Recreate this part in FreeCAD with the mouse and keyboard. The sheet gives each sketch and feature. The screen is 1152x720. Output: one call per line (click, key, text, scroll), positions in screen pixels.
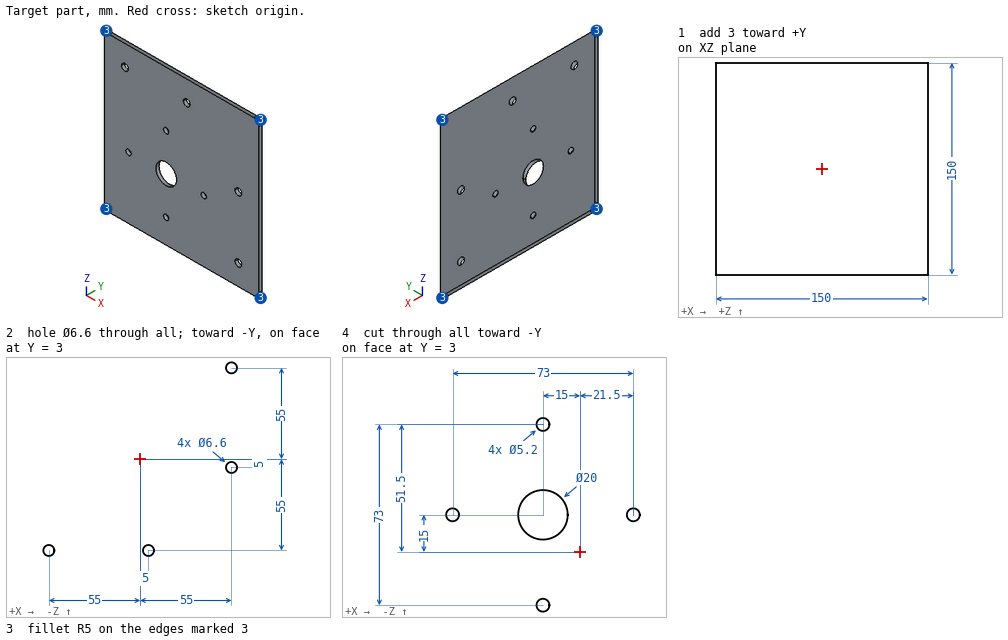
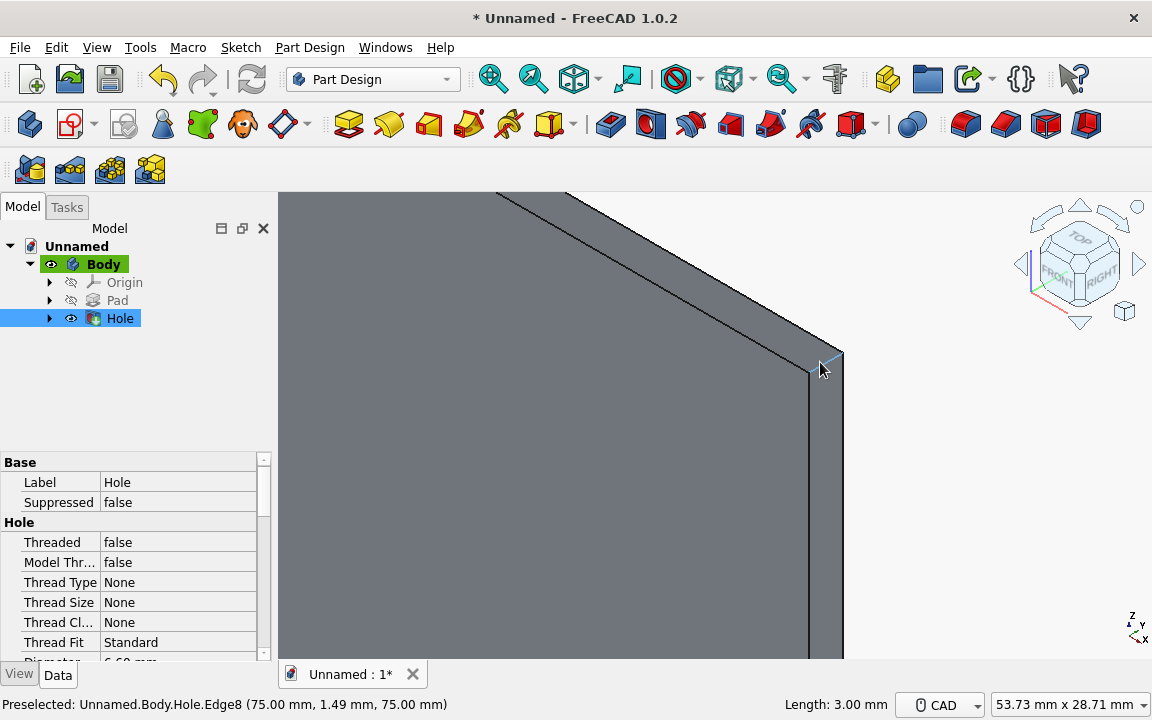
click(494, 80)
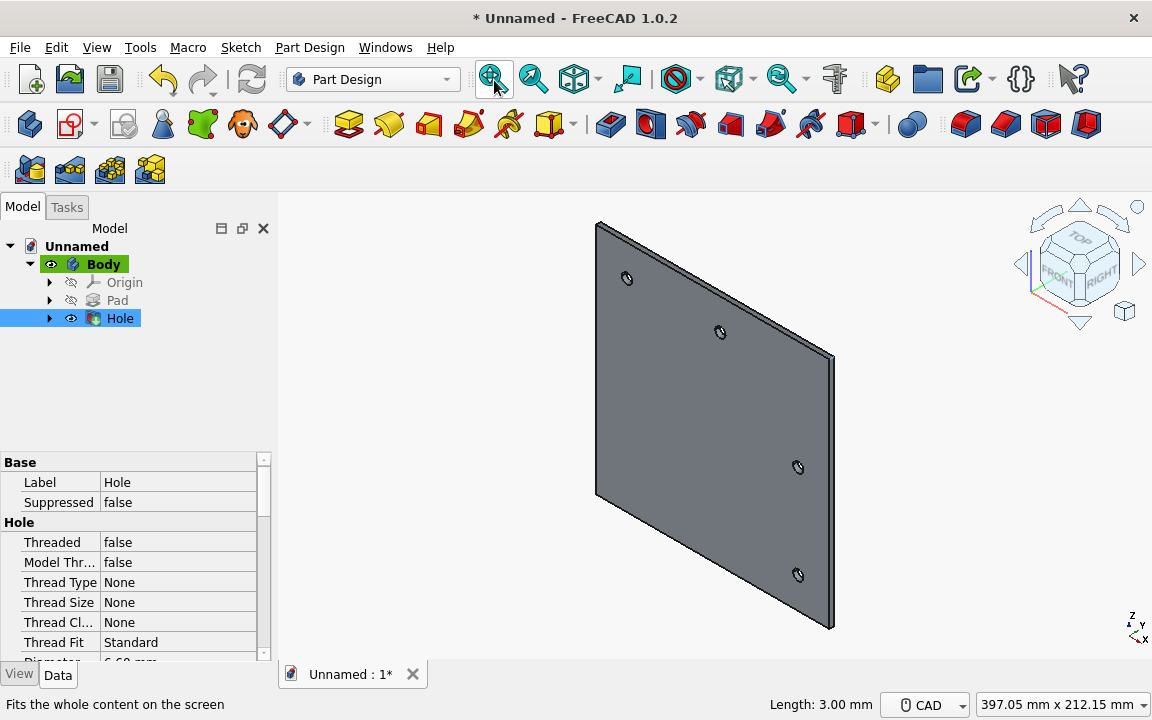
key(2)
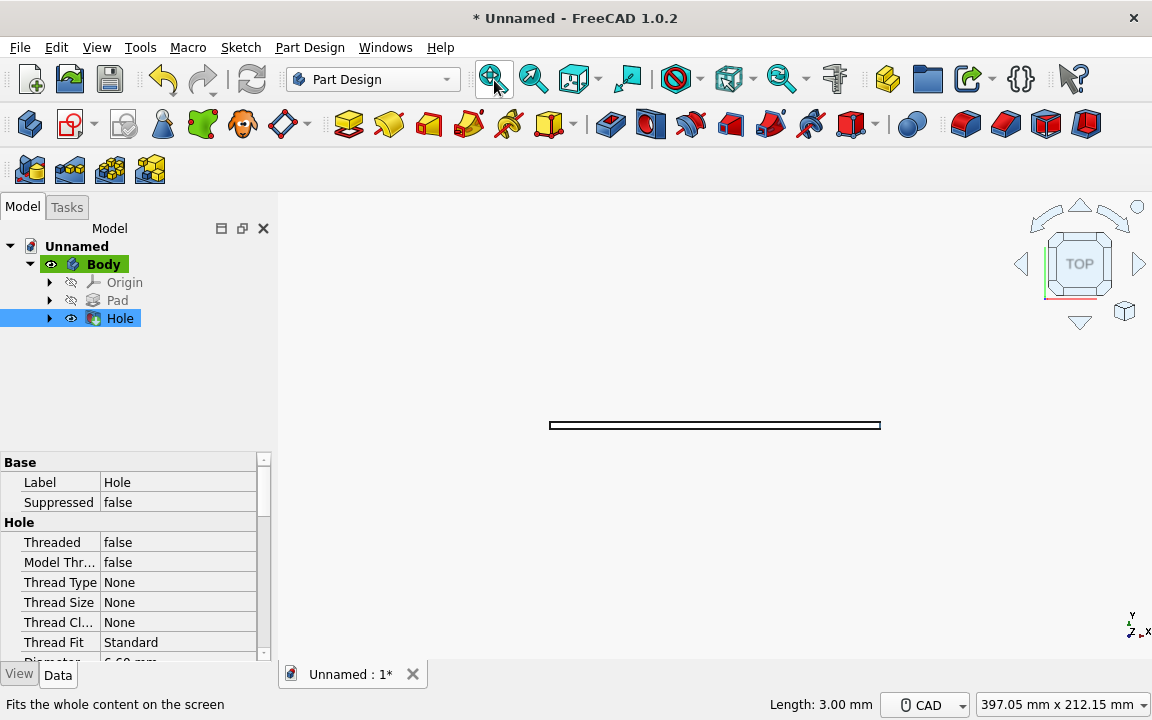
click(494, 80)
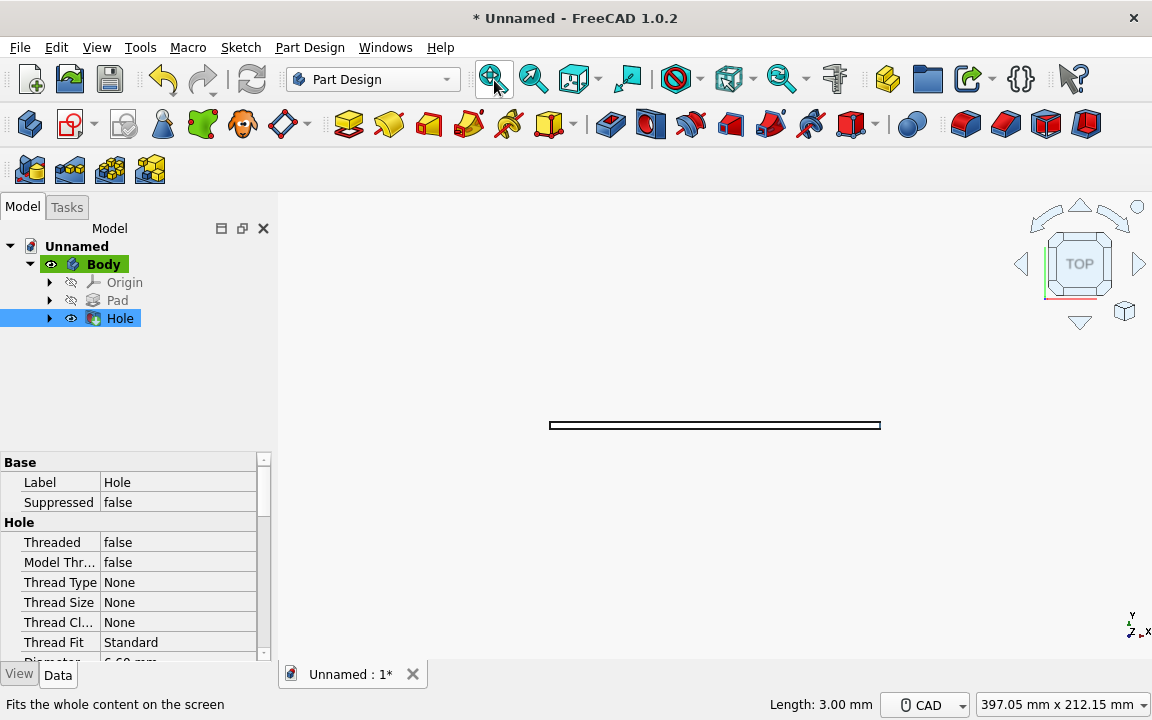
scroll(550, 424, up, 10)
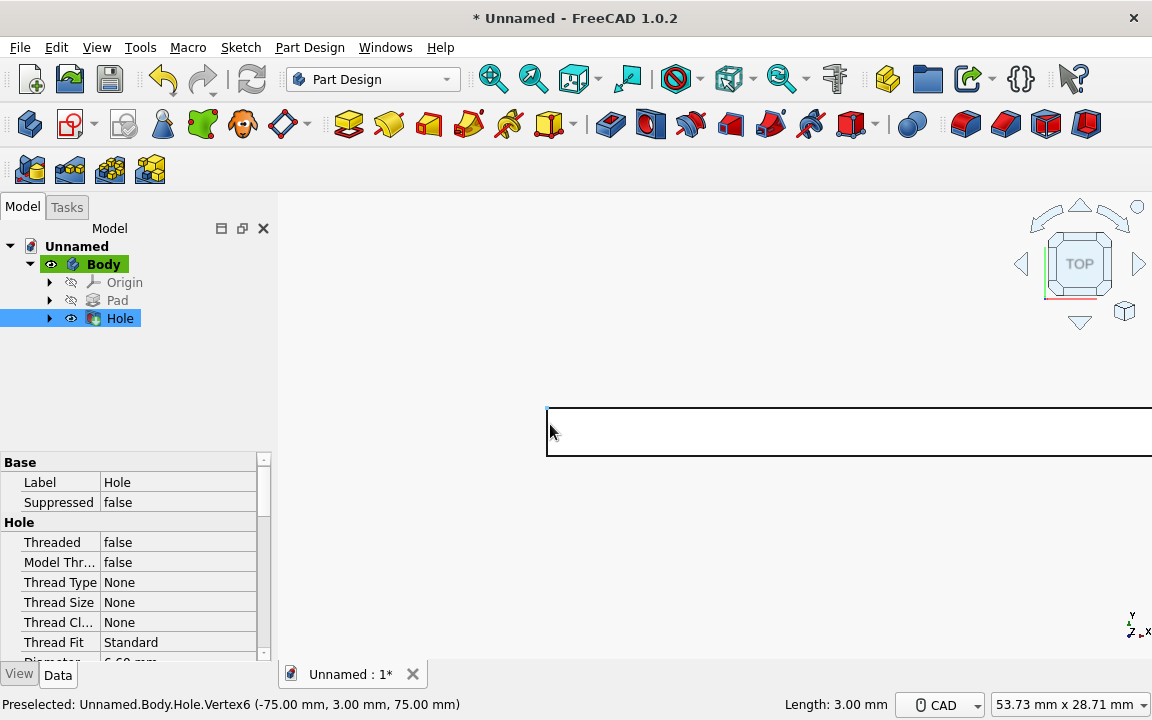
click(547, 431, ctrl)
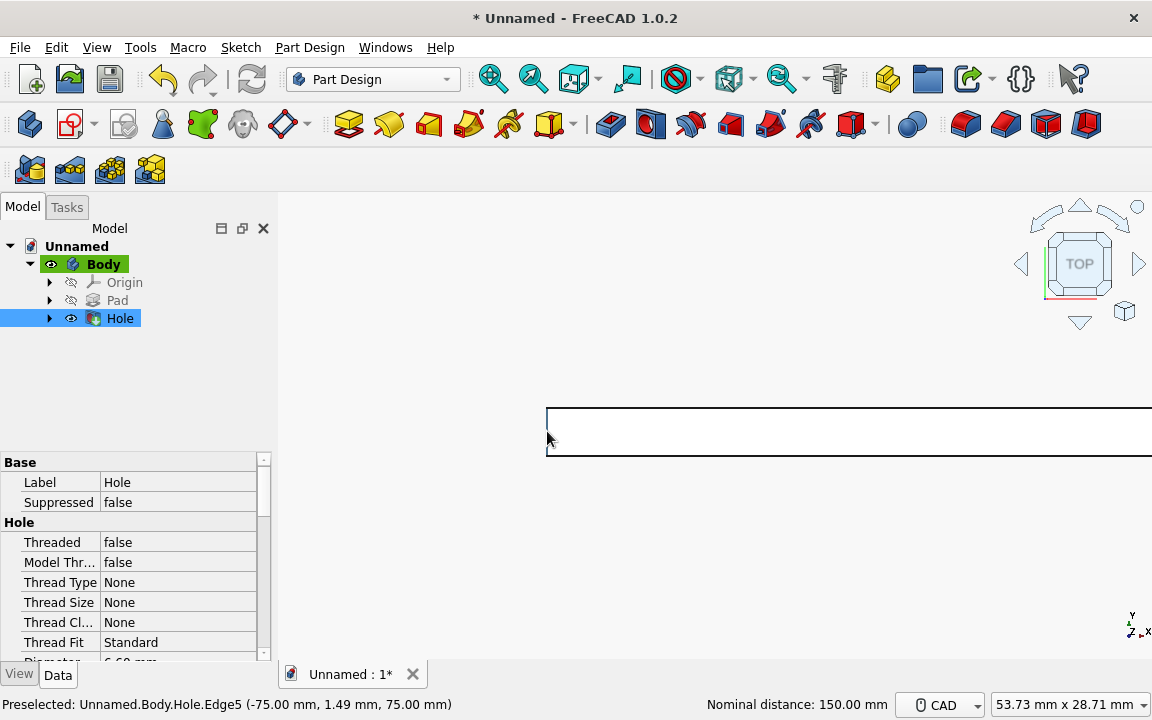
click(494, 80)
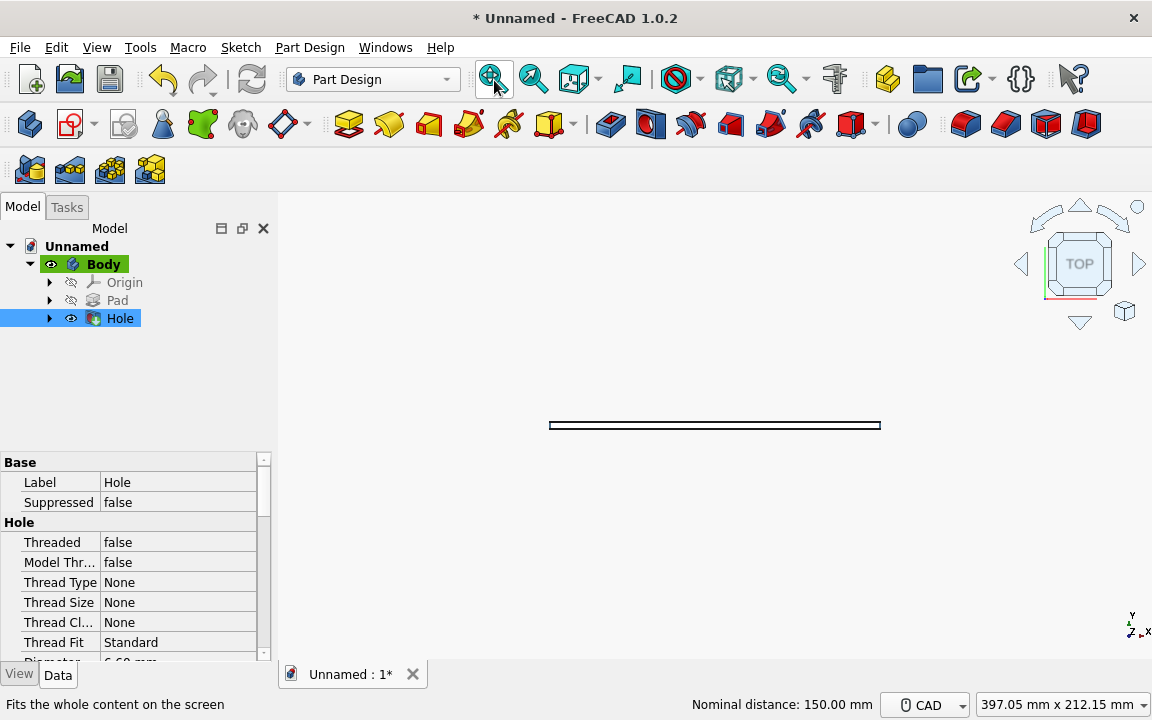
key(1)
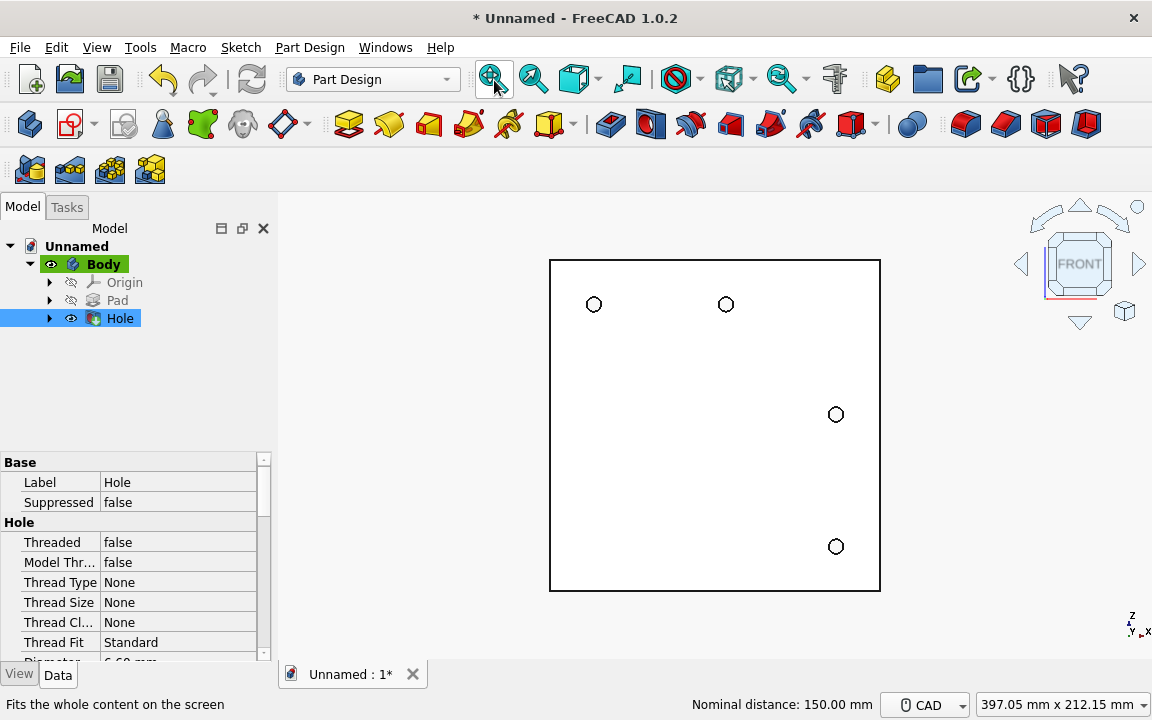
scroll(550, 590, up, 10)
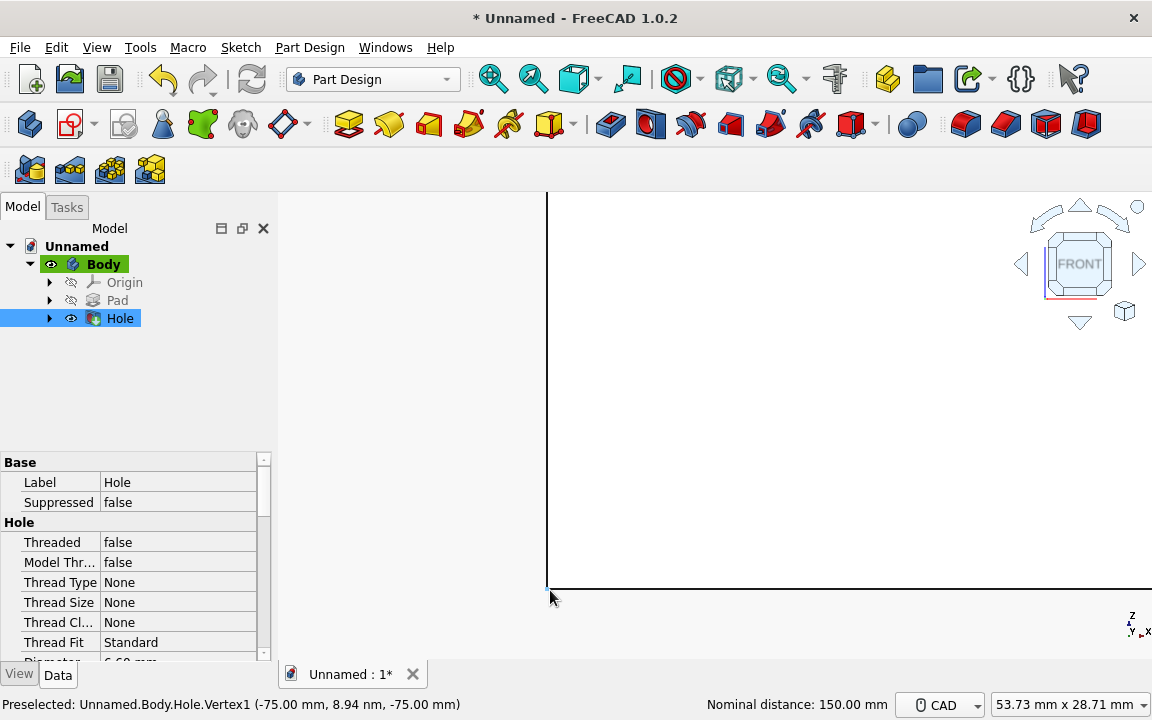
click(494, 80)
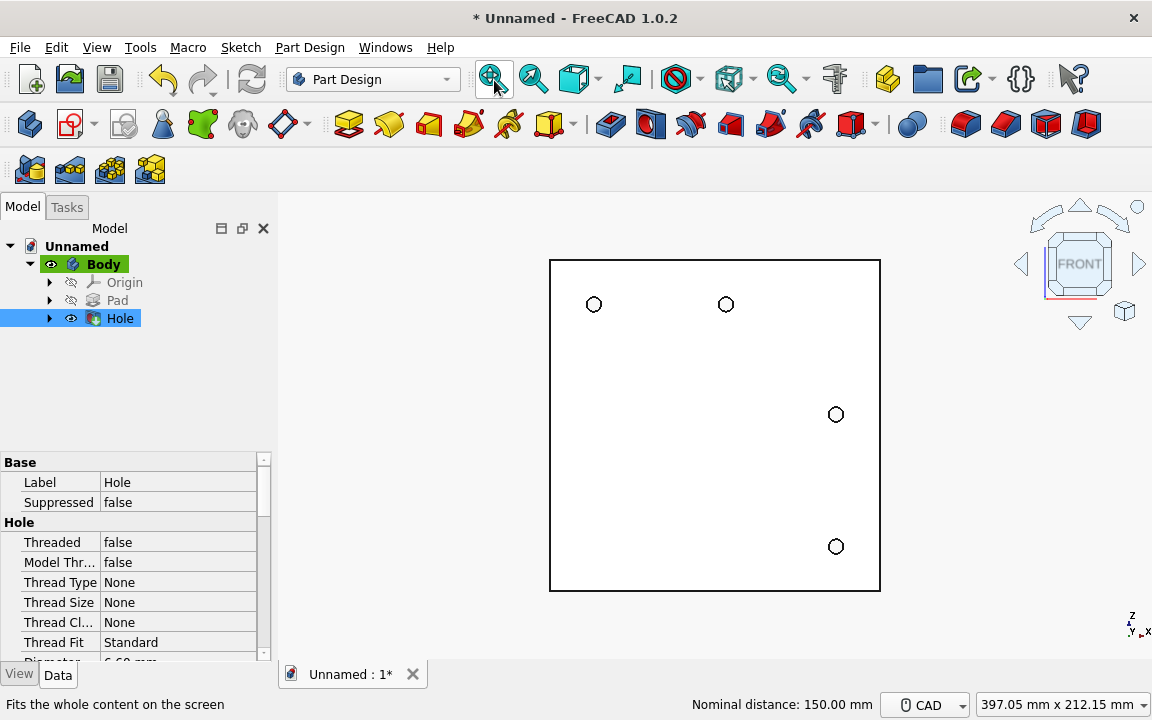
key(3)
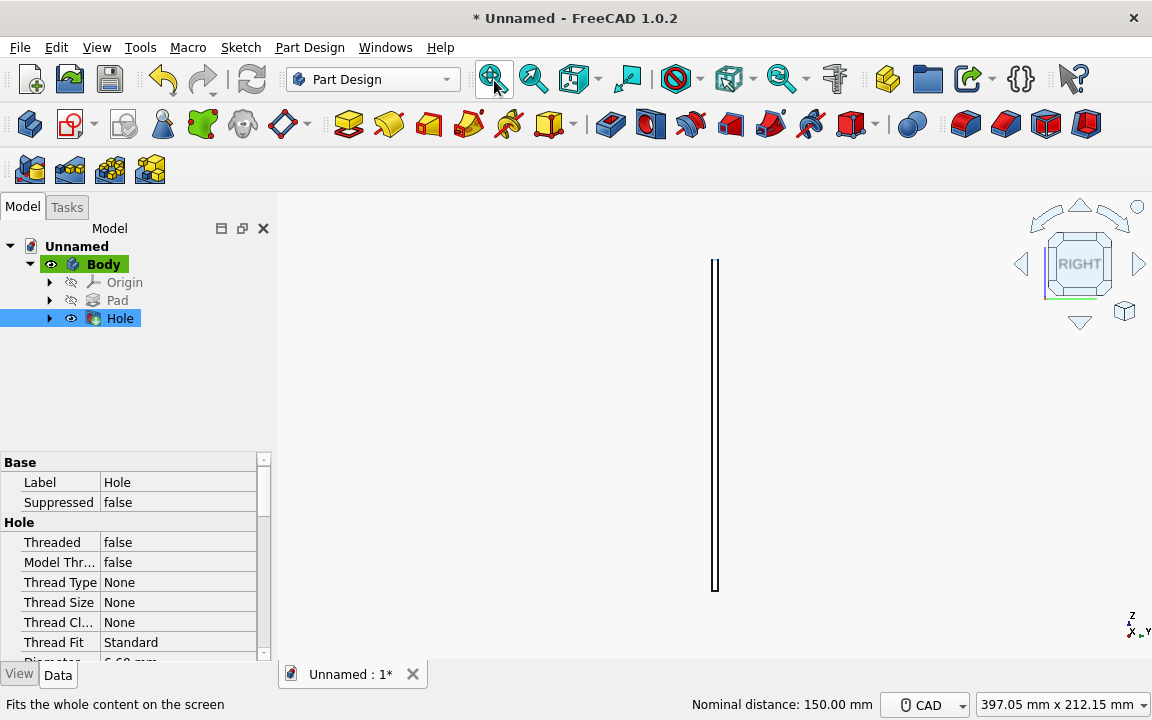
scroll(715, 590, up, 10)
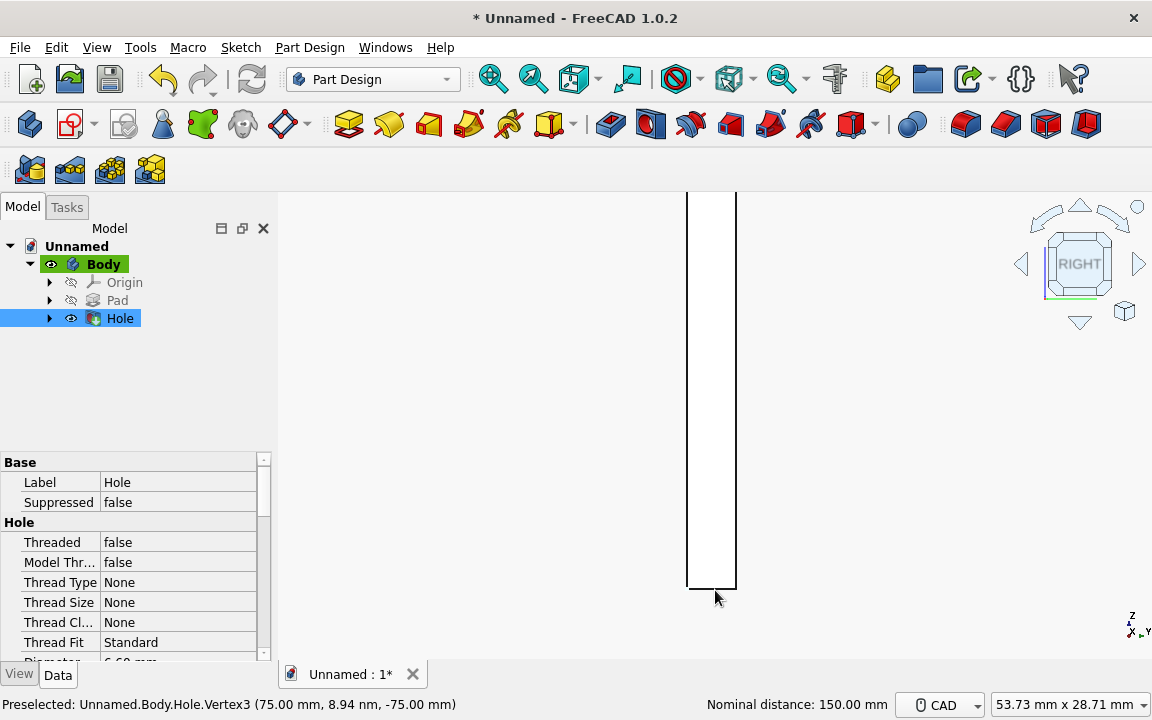
click(712, 588, ctrl)